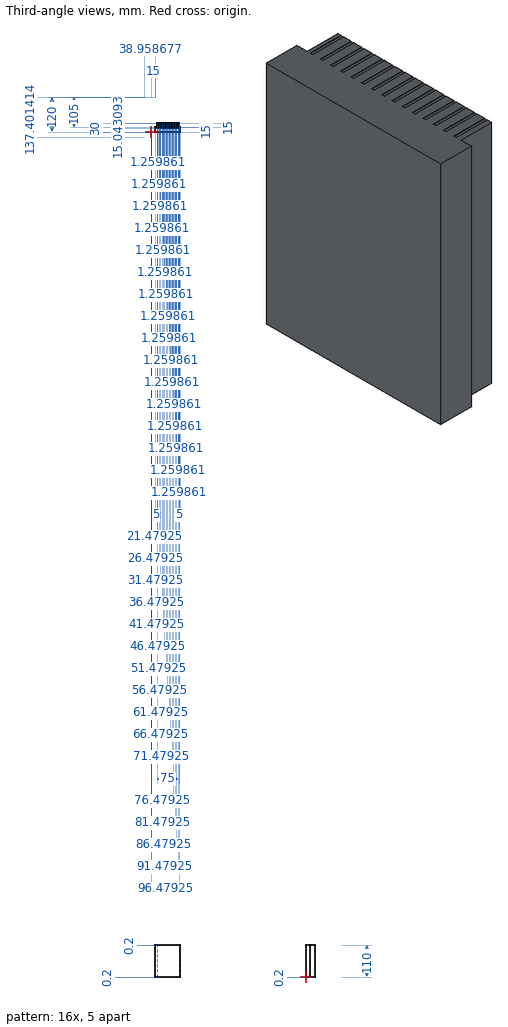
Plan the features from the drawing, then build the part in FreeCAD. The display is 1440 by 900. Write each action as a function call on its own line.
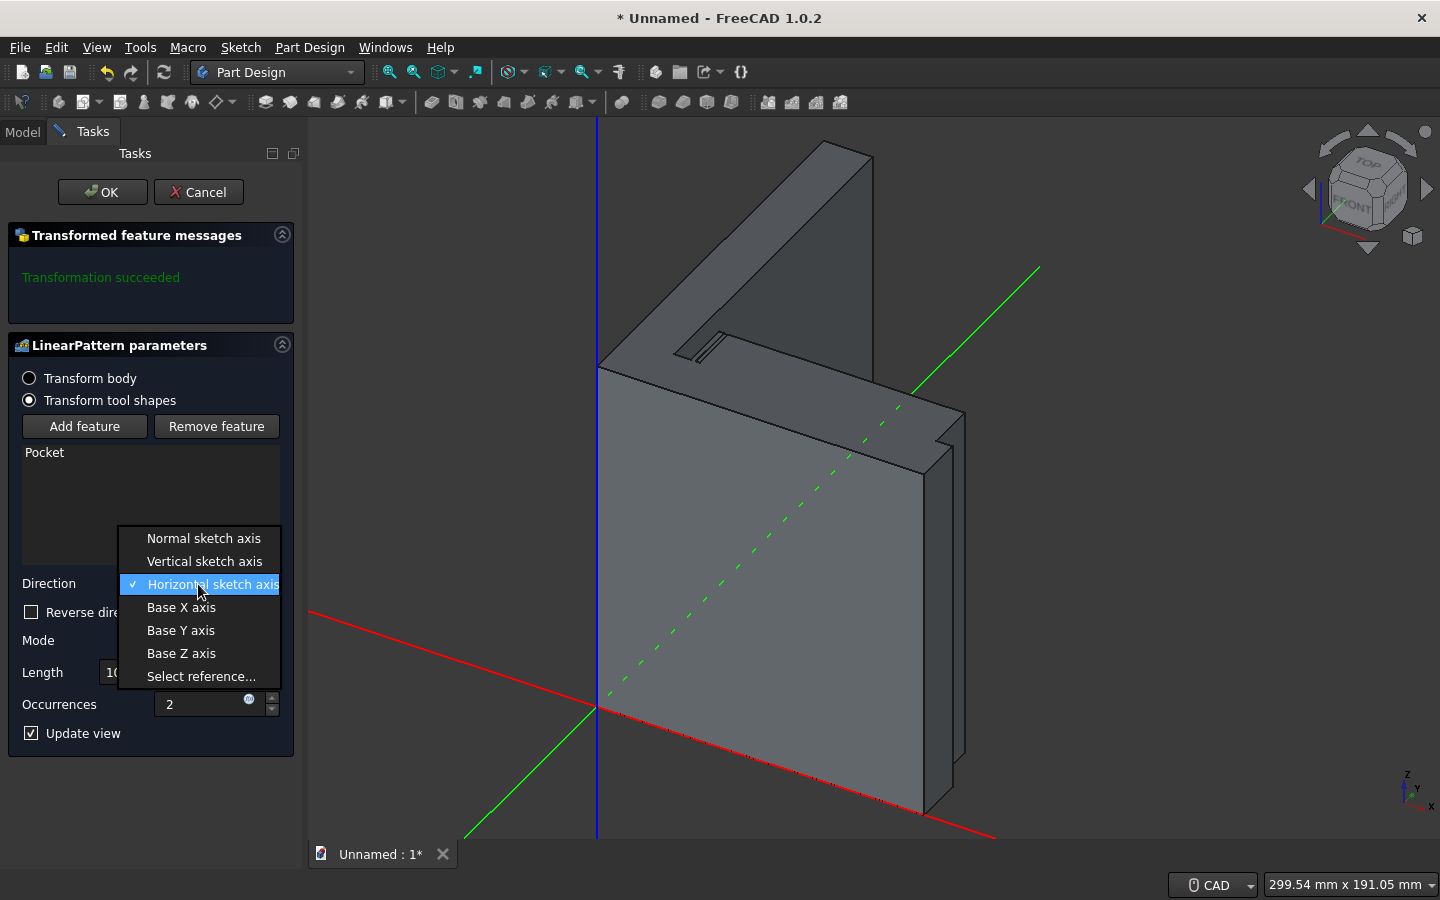
click(198, 608)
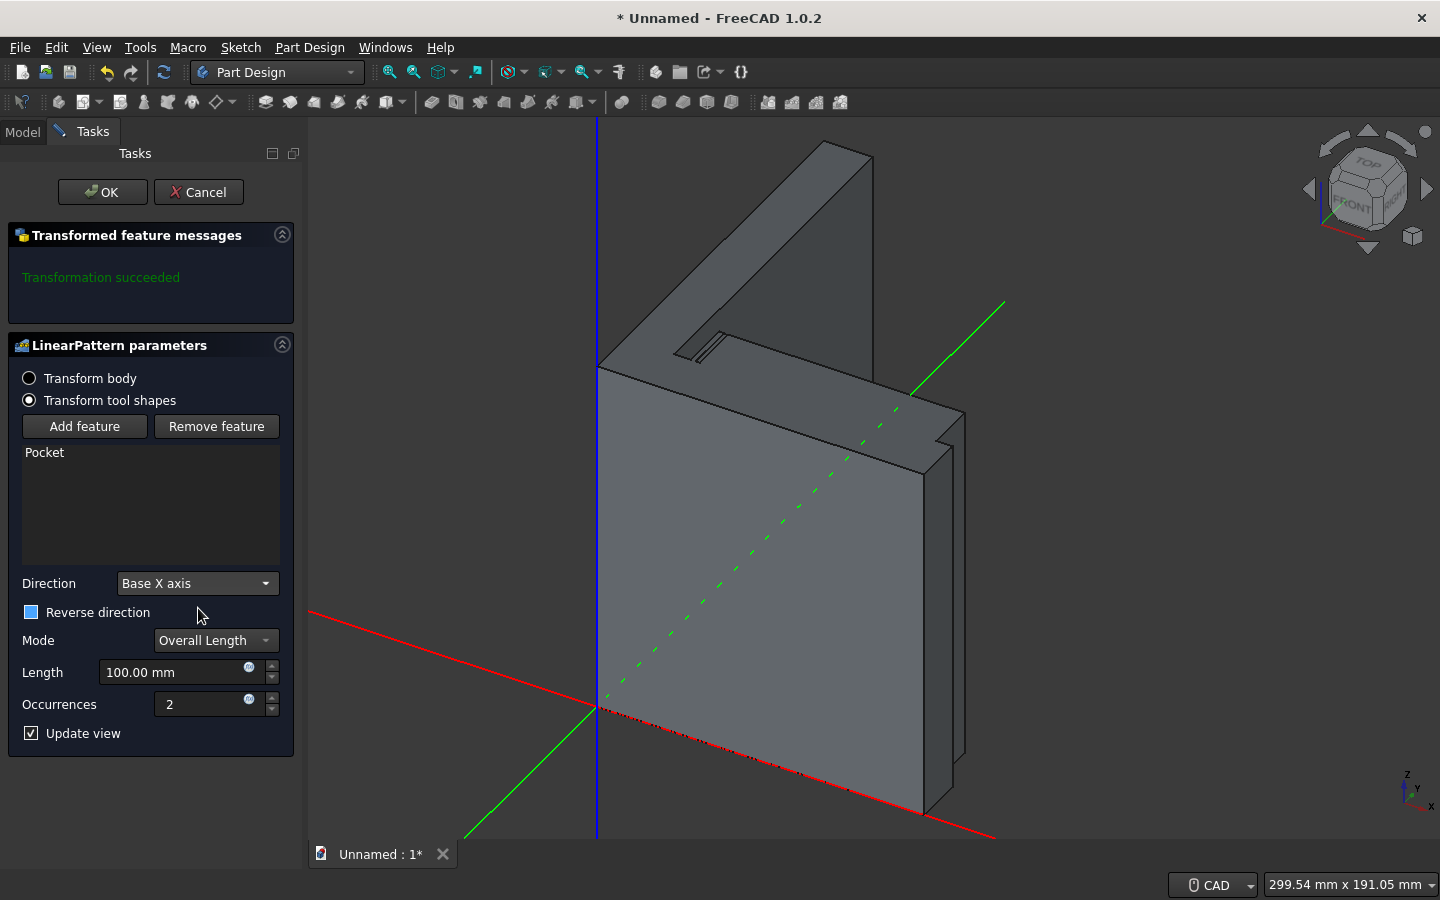
click(217, 640)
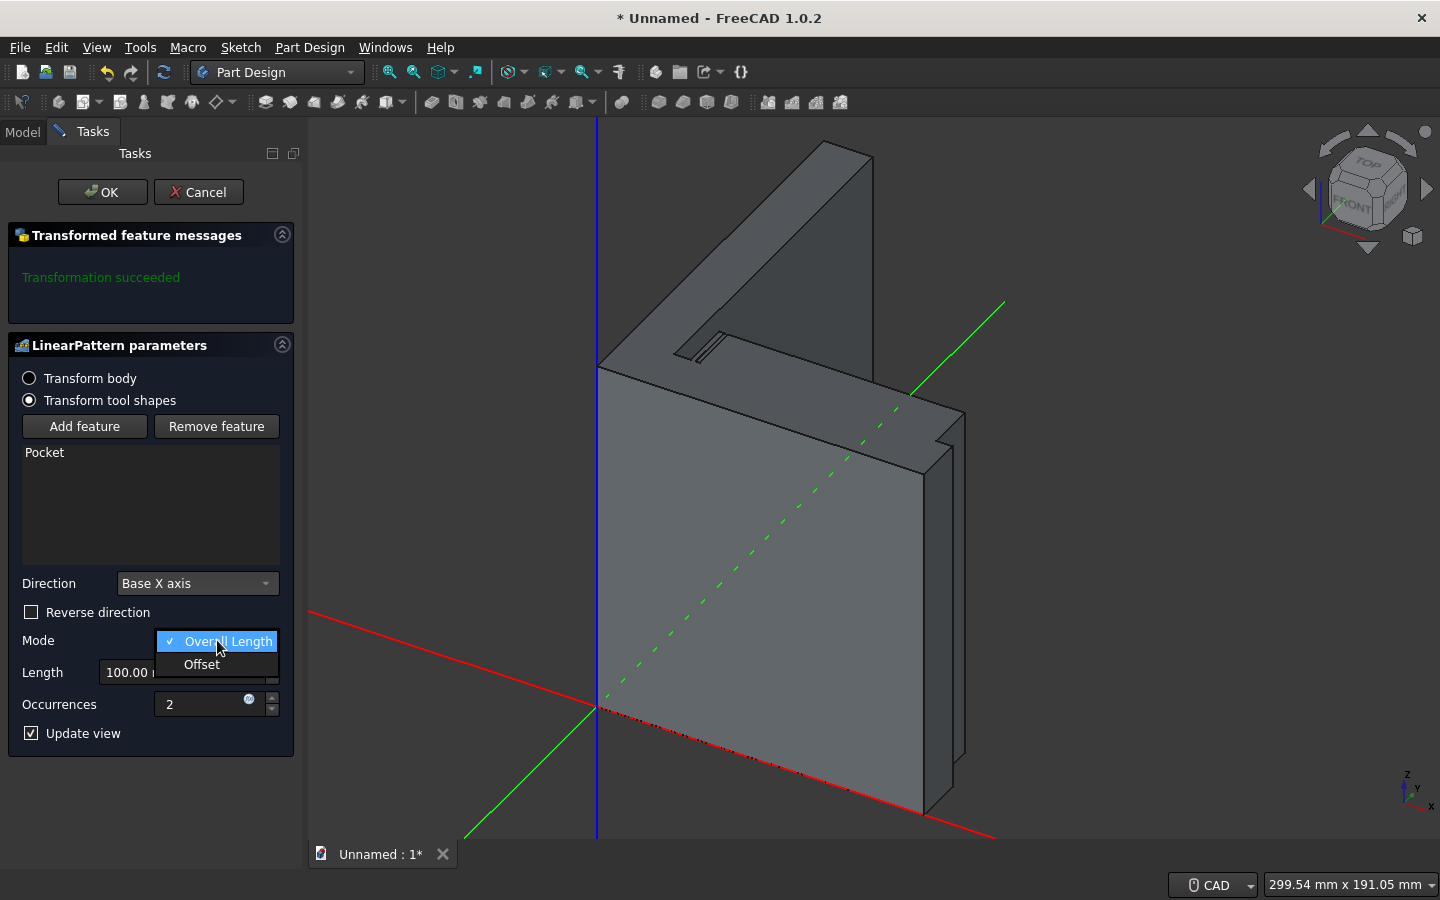
click(216, 664)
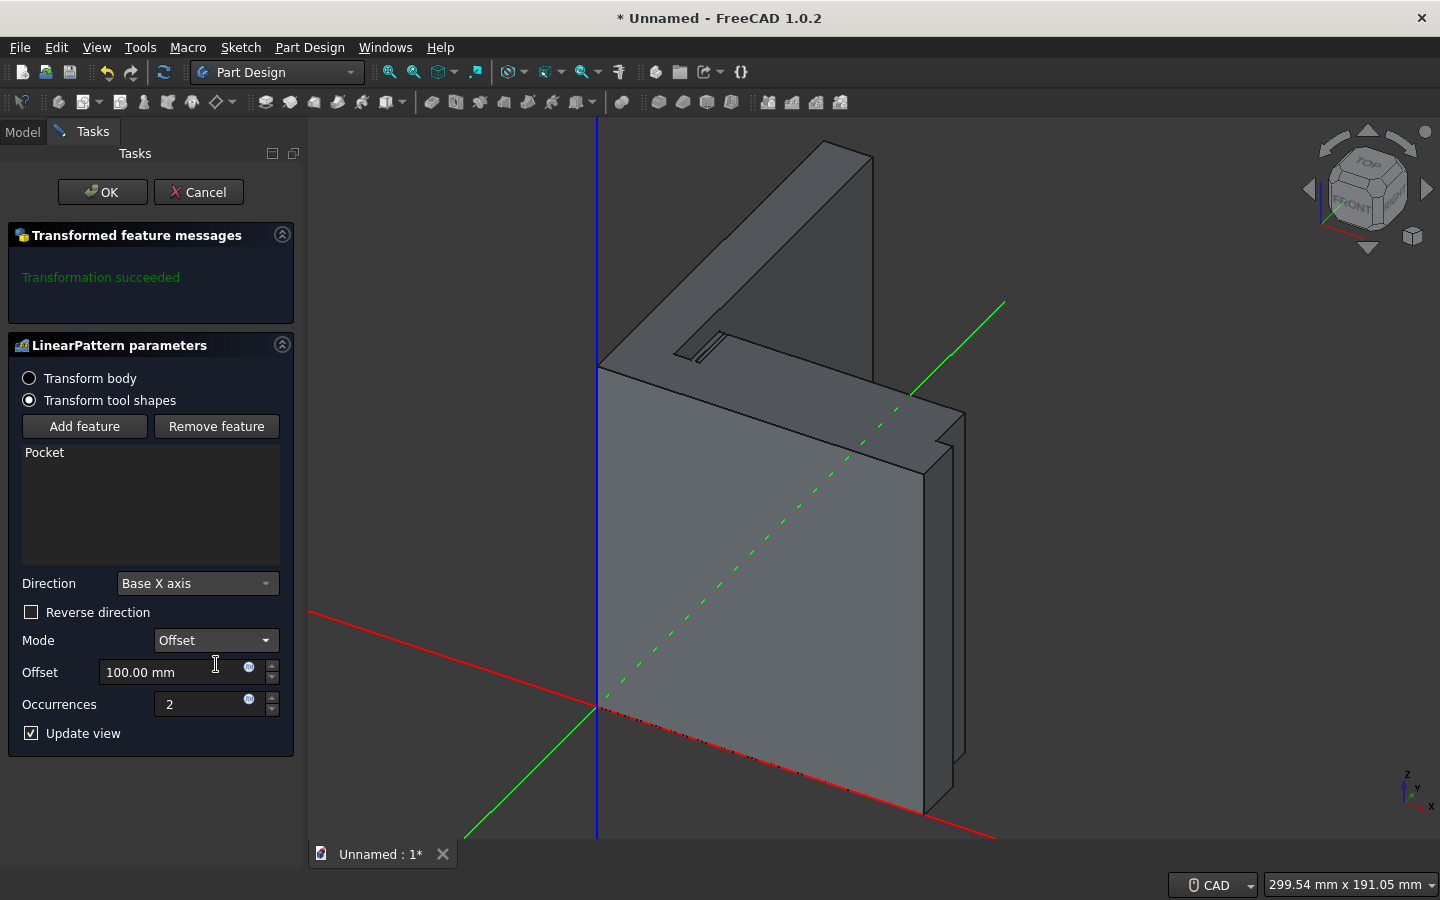
triple_click(182, 672)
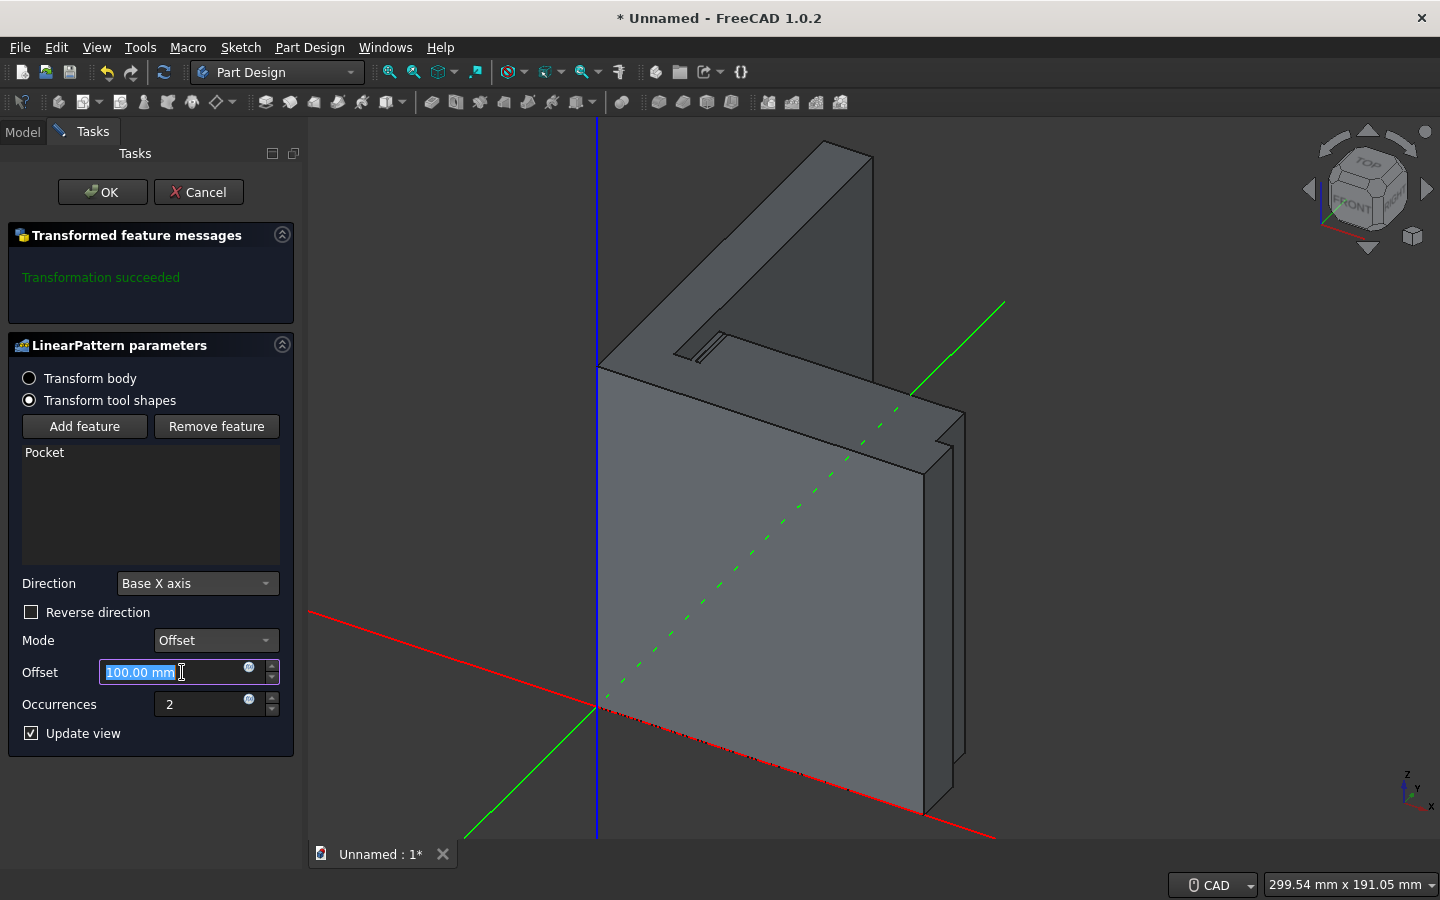
text(5)
key(Tab)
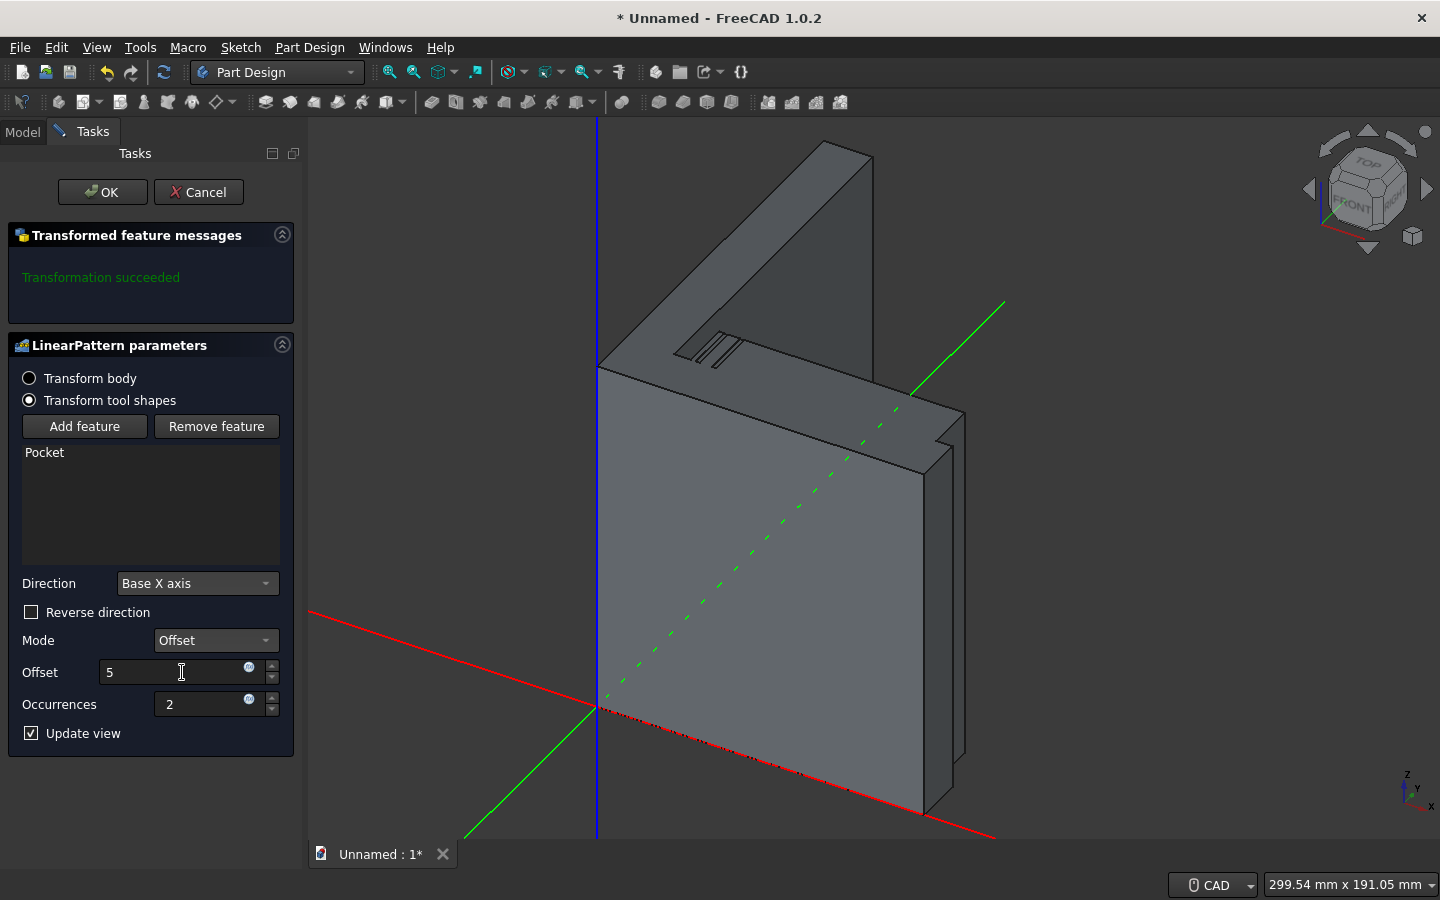
triple_click(209, 704)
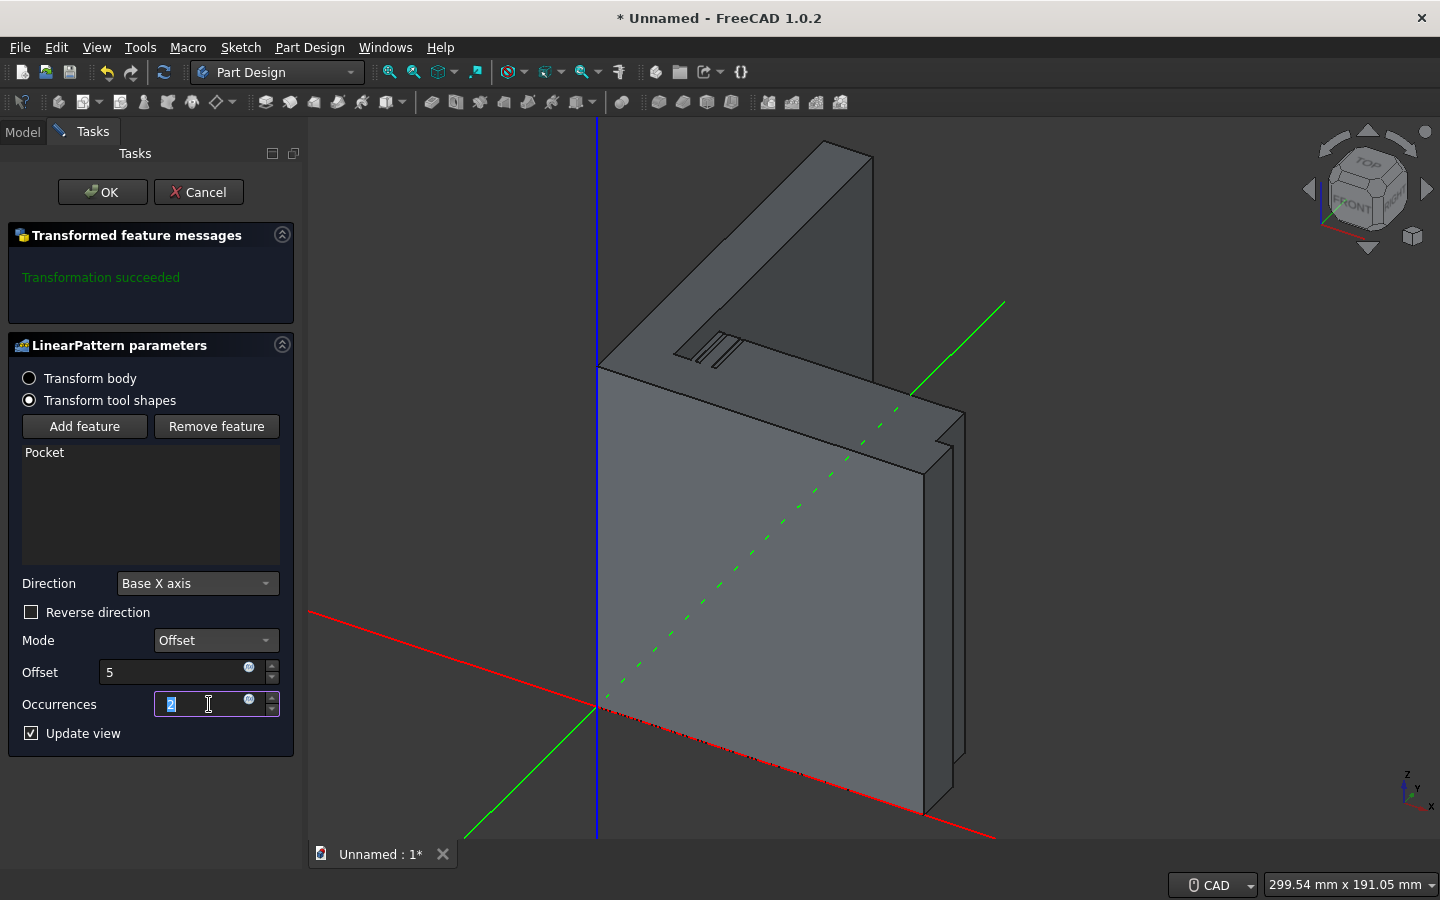
text(16)
key(Tab)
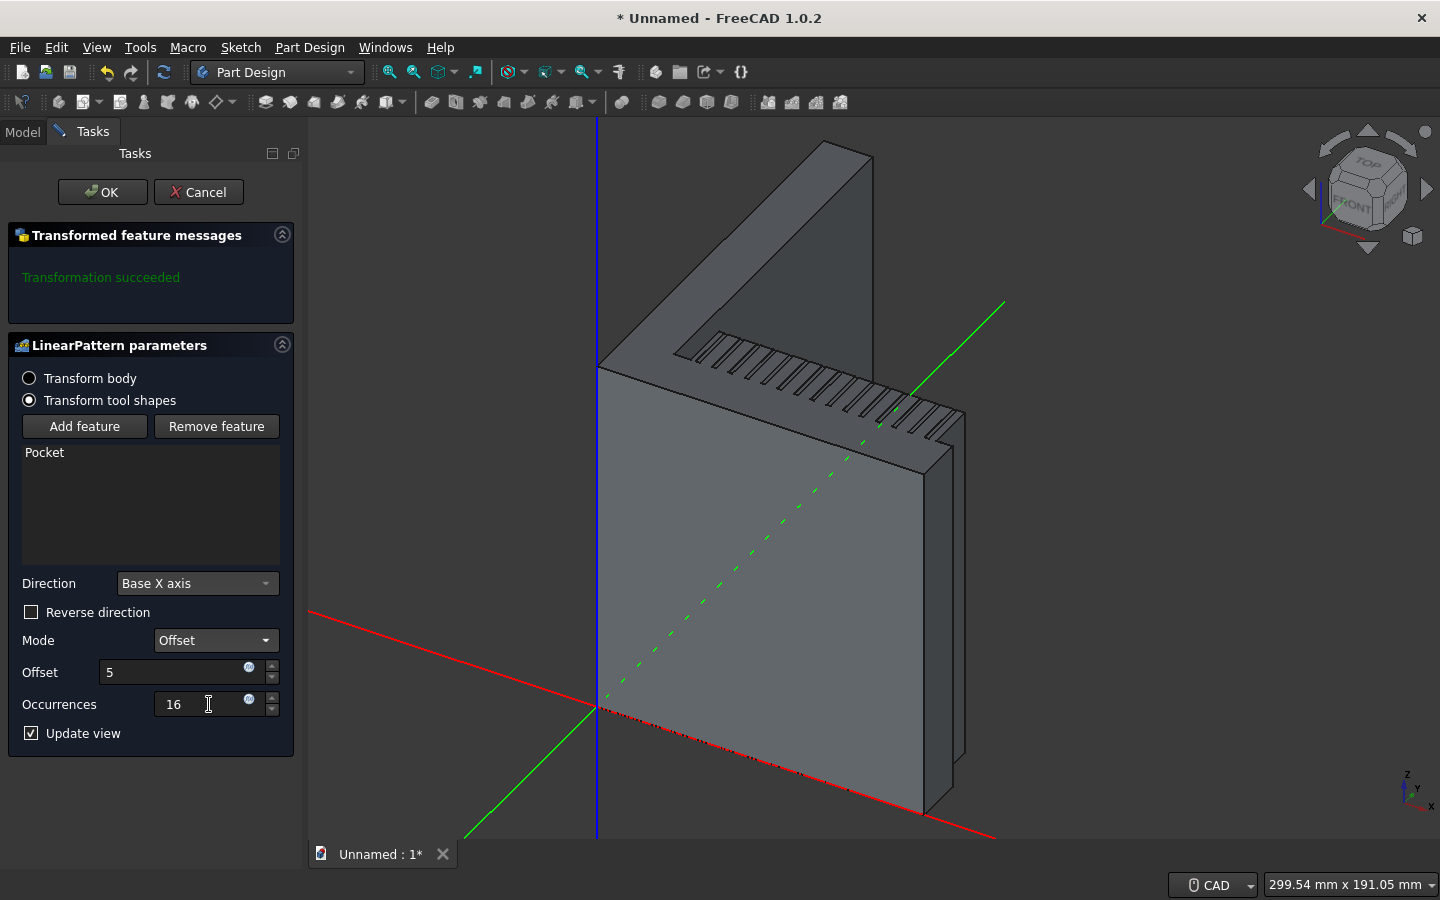
click(103, 192)